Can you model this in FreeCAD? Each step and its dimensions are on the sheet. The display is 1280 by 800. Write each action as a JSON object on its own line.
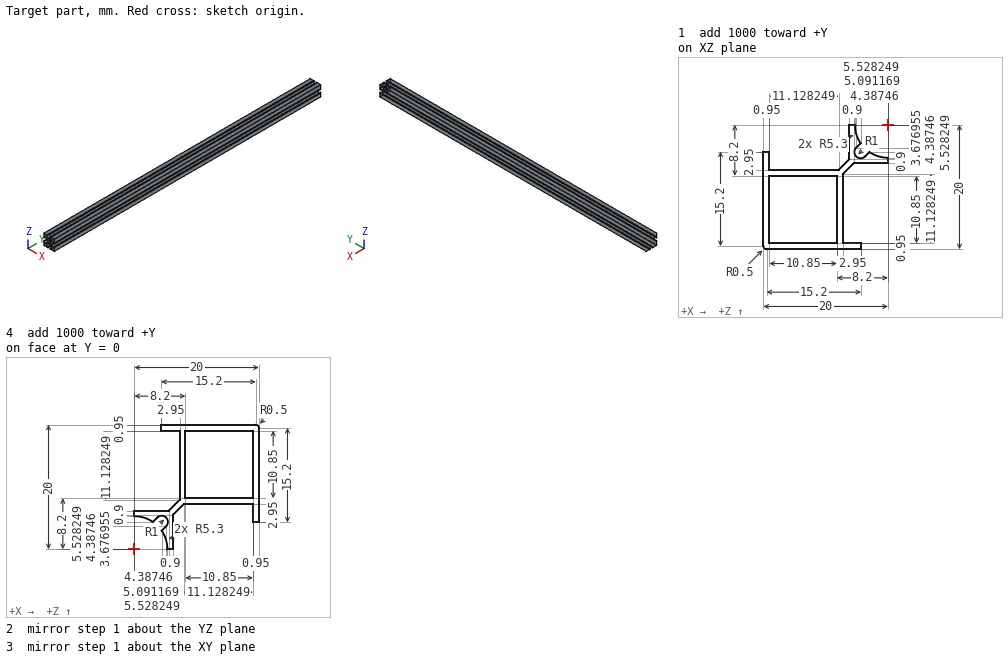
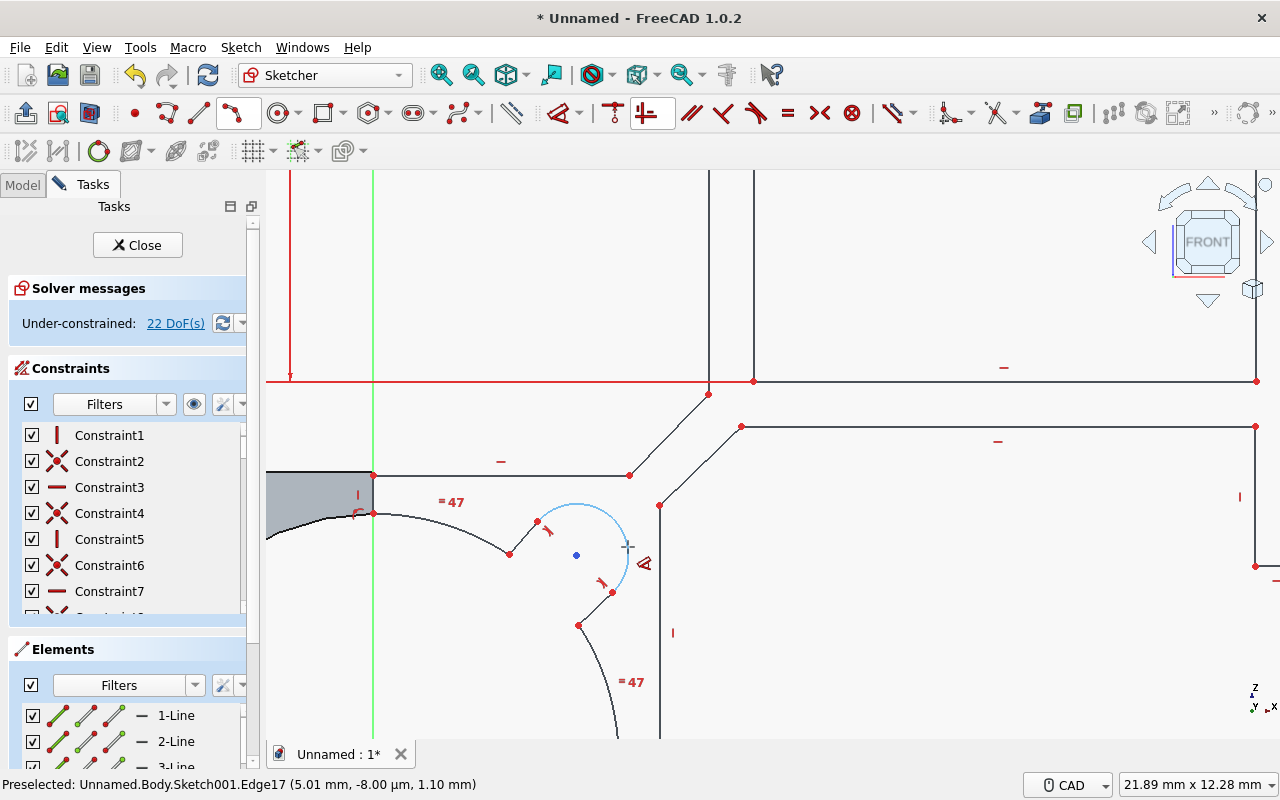
{"action": "left_click", "coordinate": [628, 547]}
{"action": "left_click", "coordinate": [643, 504]}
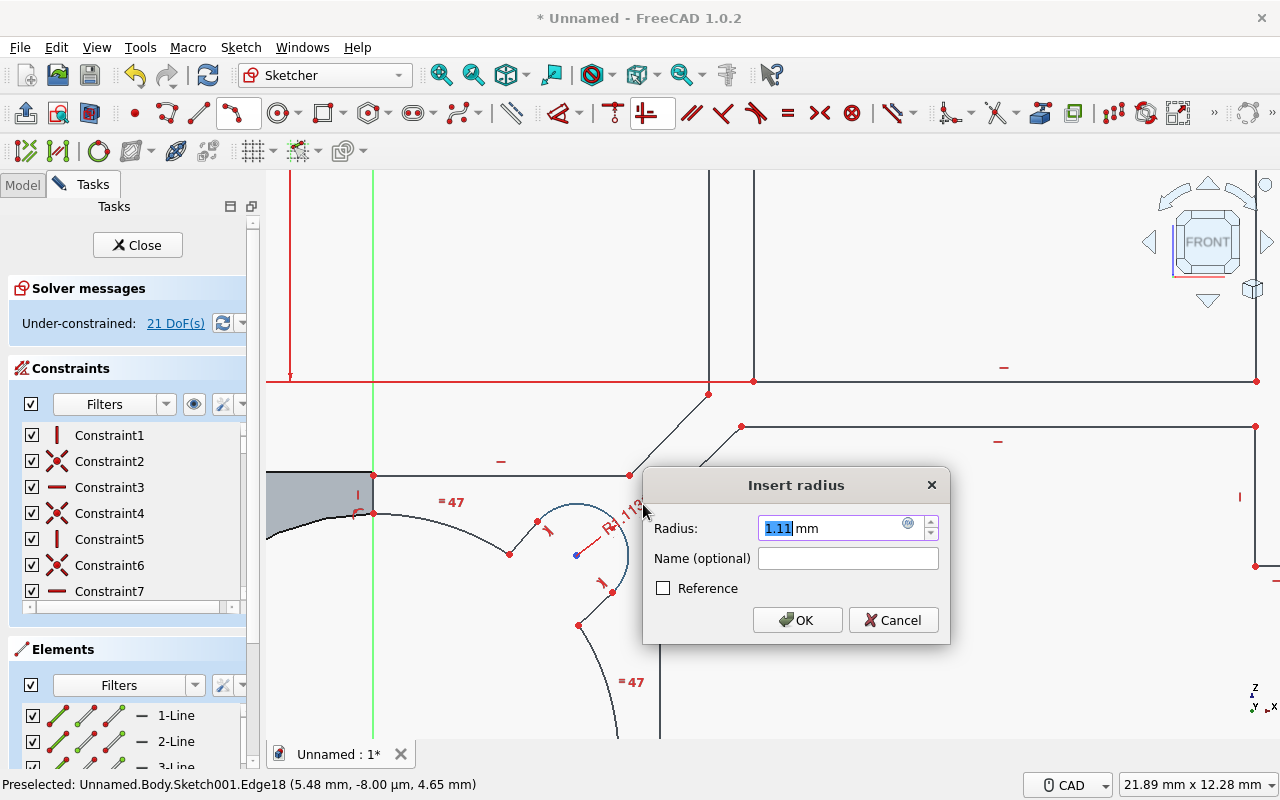
{"action": "type", "text": "1"}
{"action": "key", "text": "Return"}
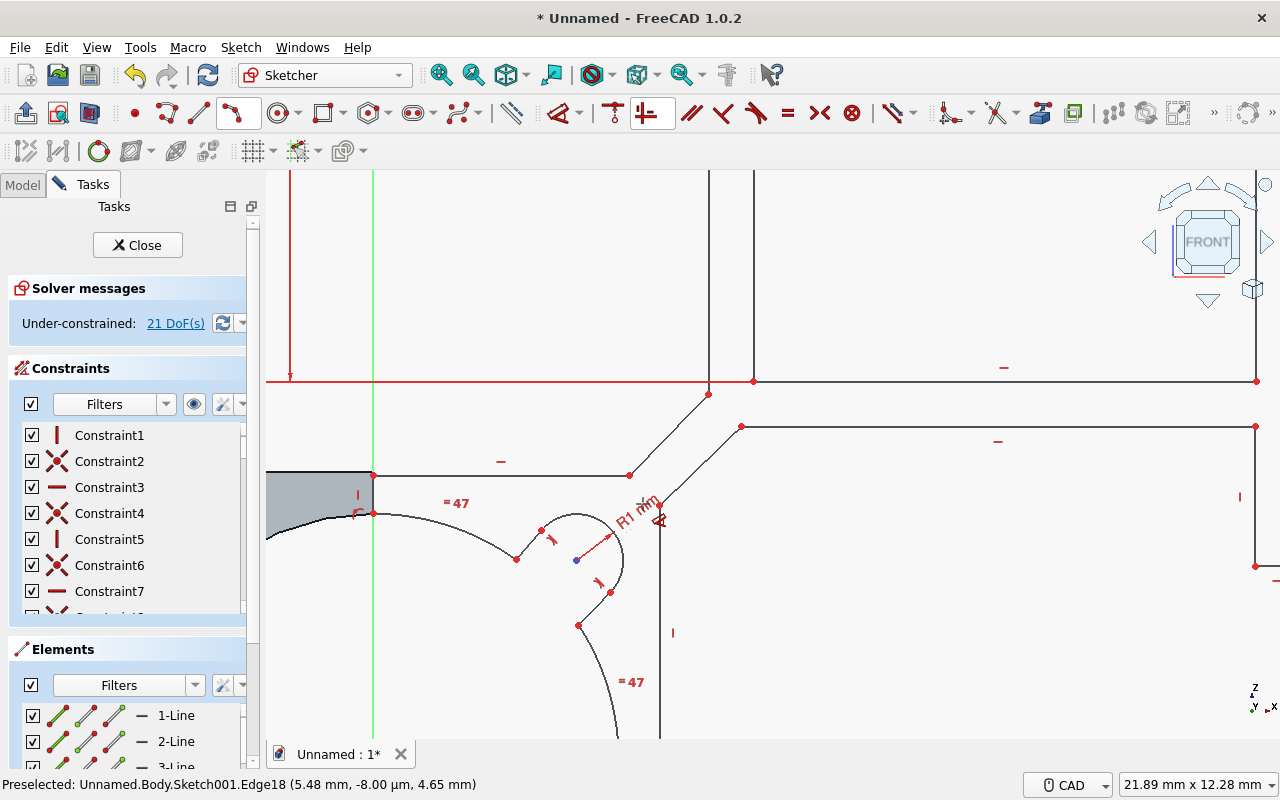
{"action": "scroll", "coordinate": [628, 547], "scroll_direction": "down", "scroll_amount": 5}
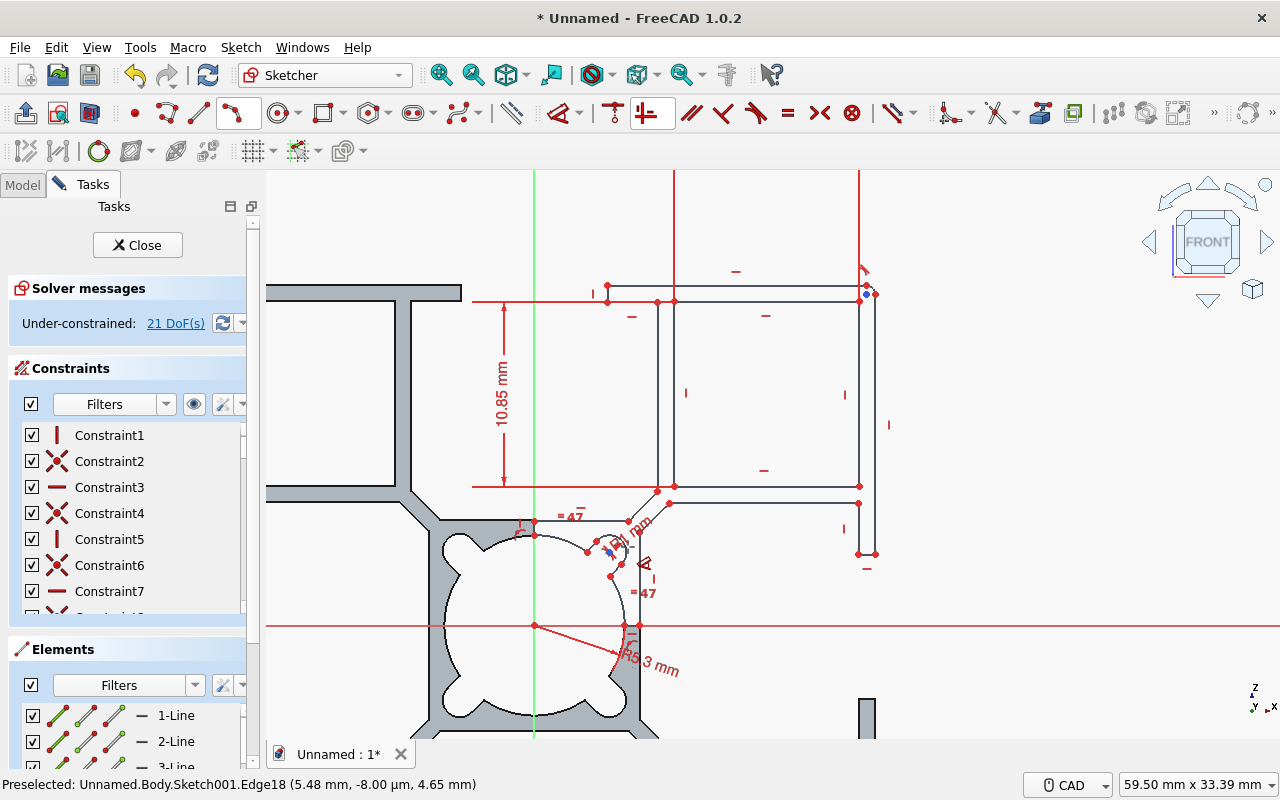
{"action": "scroll", "coordinate": [874, 291], "scroll_direction": "up", "scroll_amount": 8}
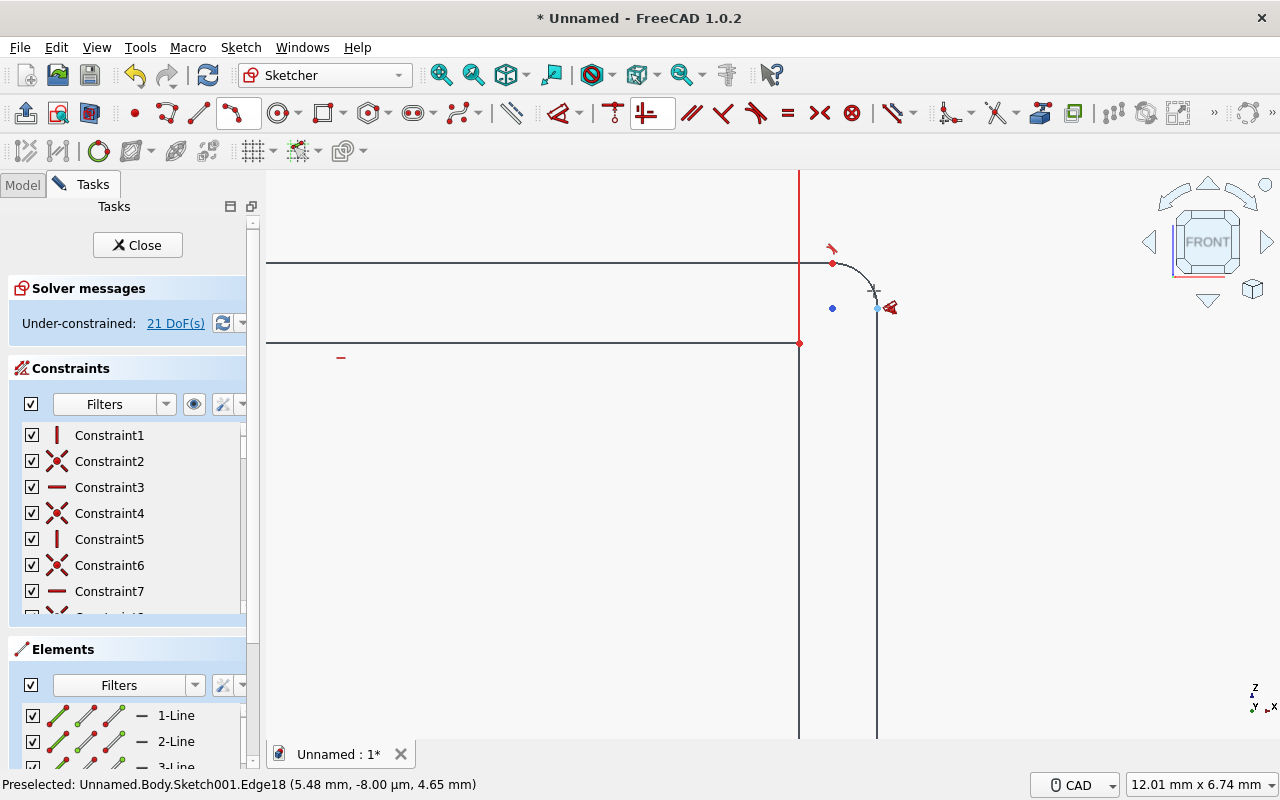
{"action": "left_click", "coordinate": [873, 288]}
{"action": "left_click", "coordinate": [902, 274]}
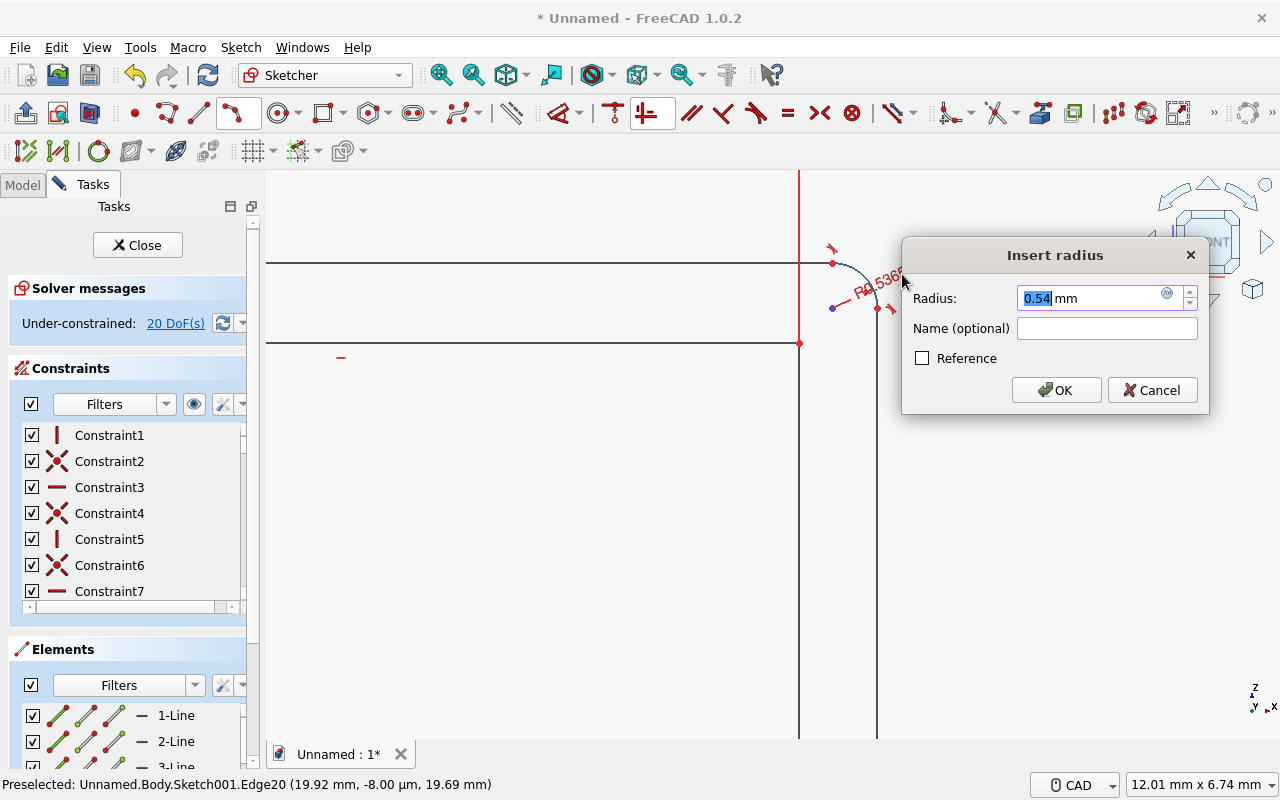
{"action": "type", "text": "0.5"}
{"action": "key", "text": "Return"}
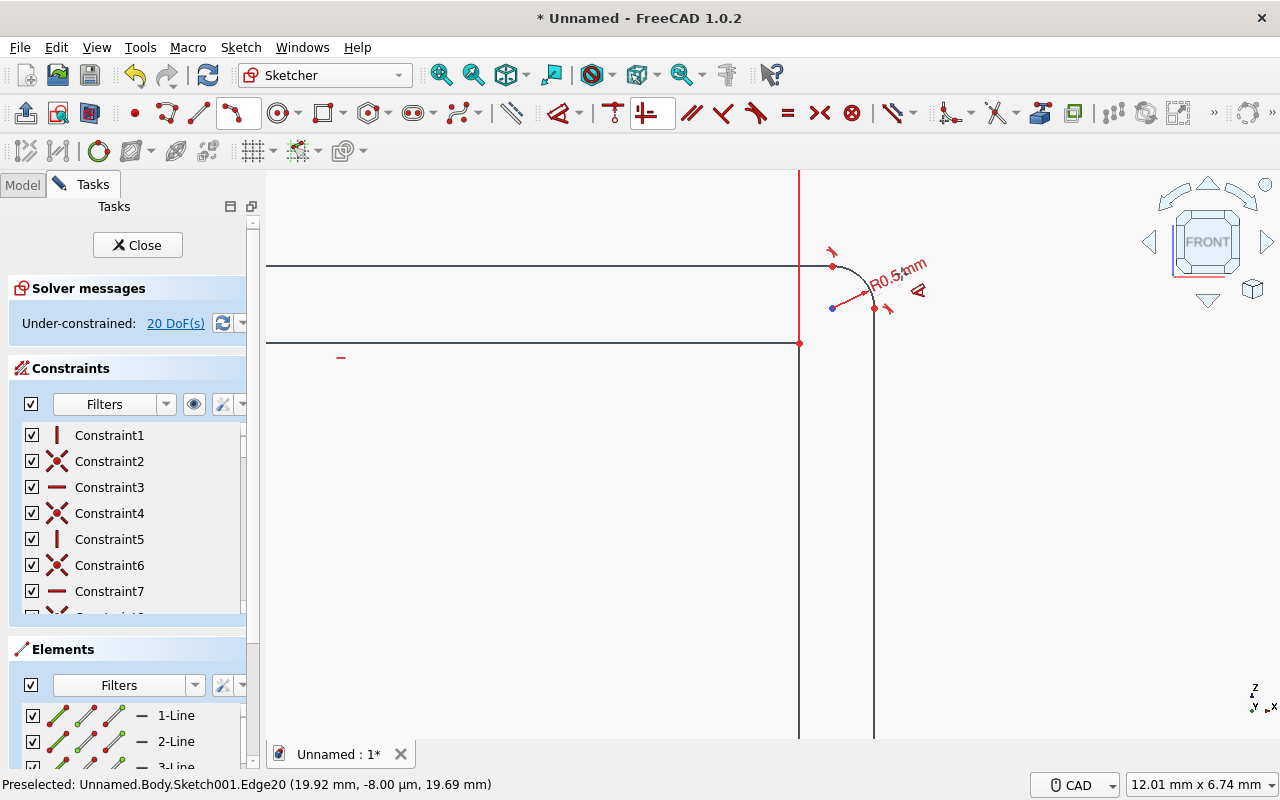
{"action": "scroll", "coordinate": [874, 290], "scroll_direction": "down", "scroll_amount": 8}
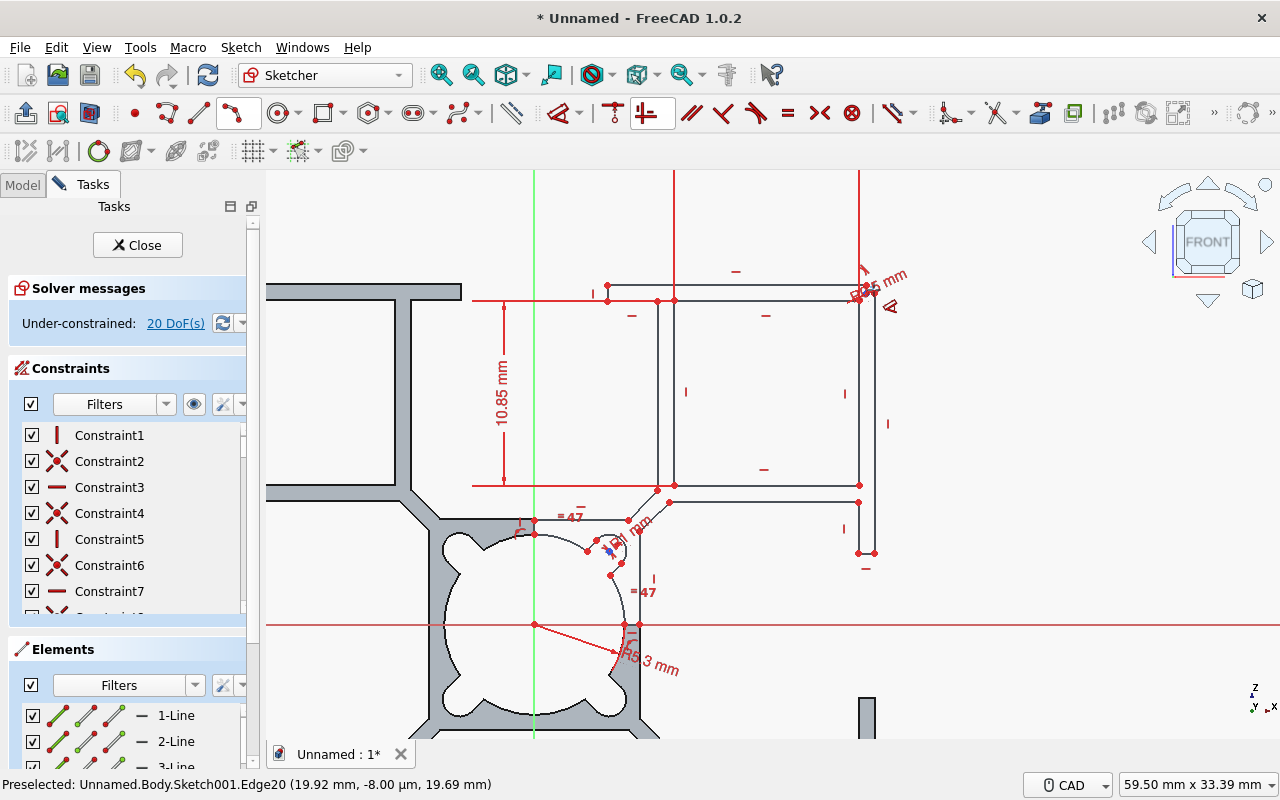
{"action": "scroll", "coordinate": [635, 625], "scroll_direction": "up", "scroll_amount": 6}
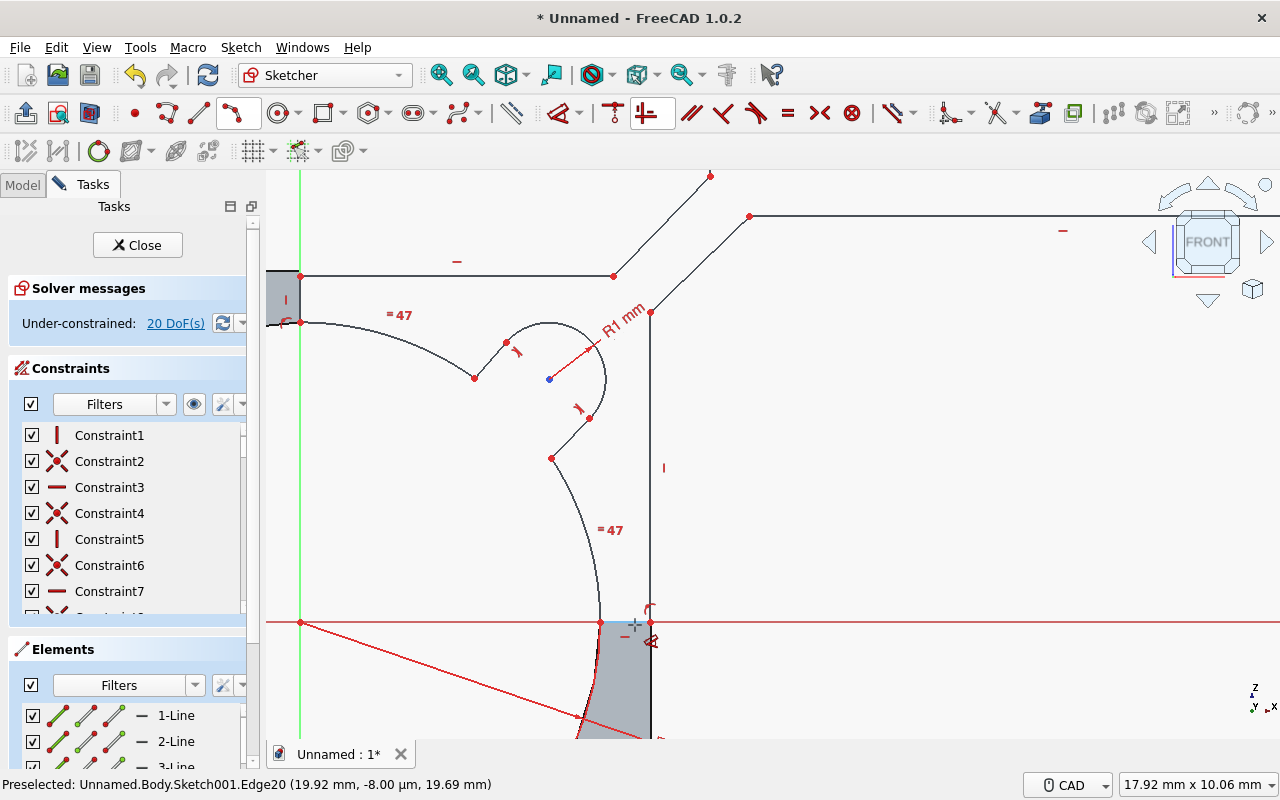
{"action": "left_click", "coordinate": [635, 622]}
{"action": "left_click", "coordinate": [625, 656]}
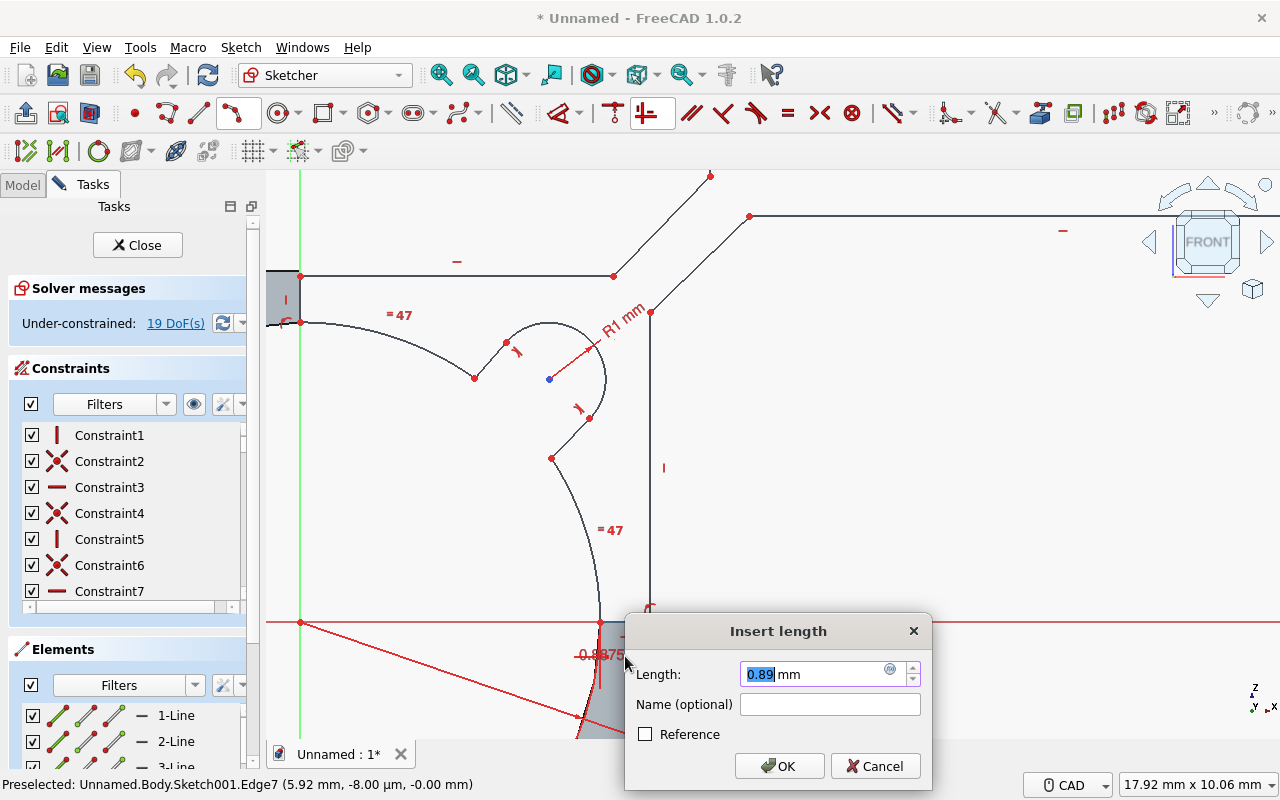
{"action": "type", "text": "0.9"}
{"action": "key", "text": "Return"}